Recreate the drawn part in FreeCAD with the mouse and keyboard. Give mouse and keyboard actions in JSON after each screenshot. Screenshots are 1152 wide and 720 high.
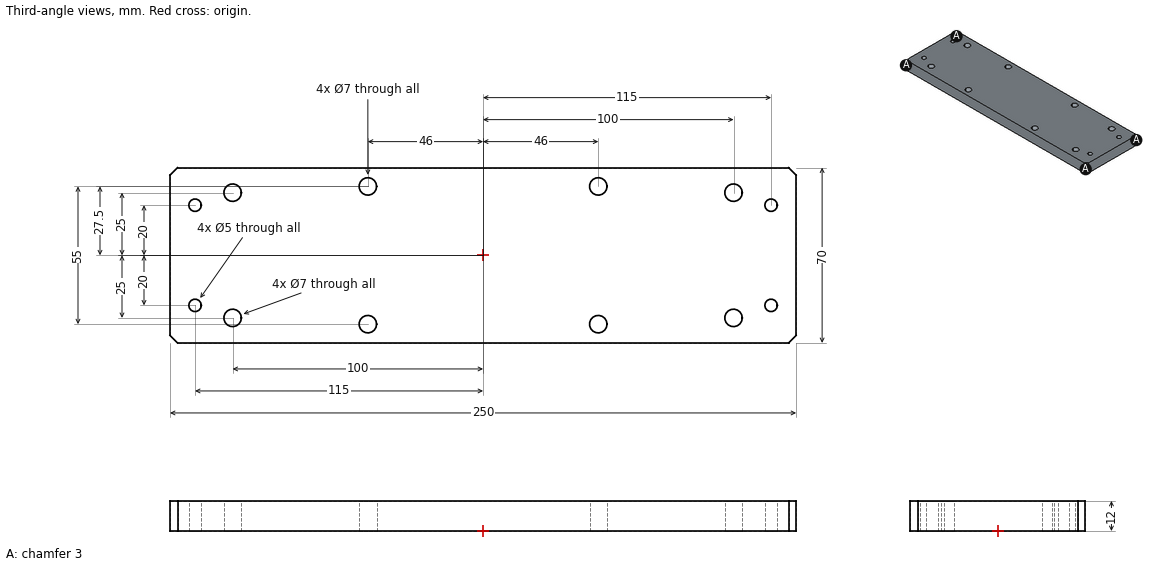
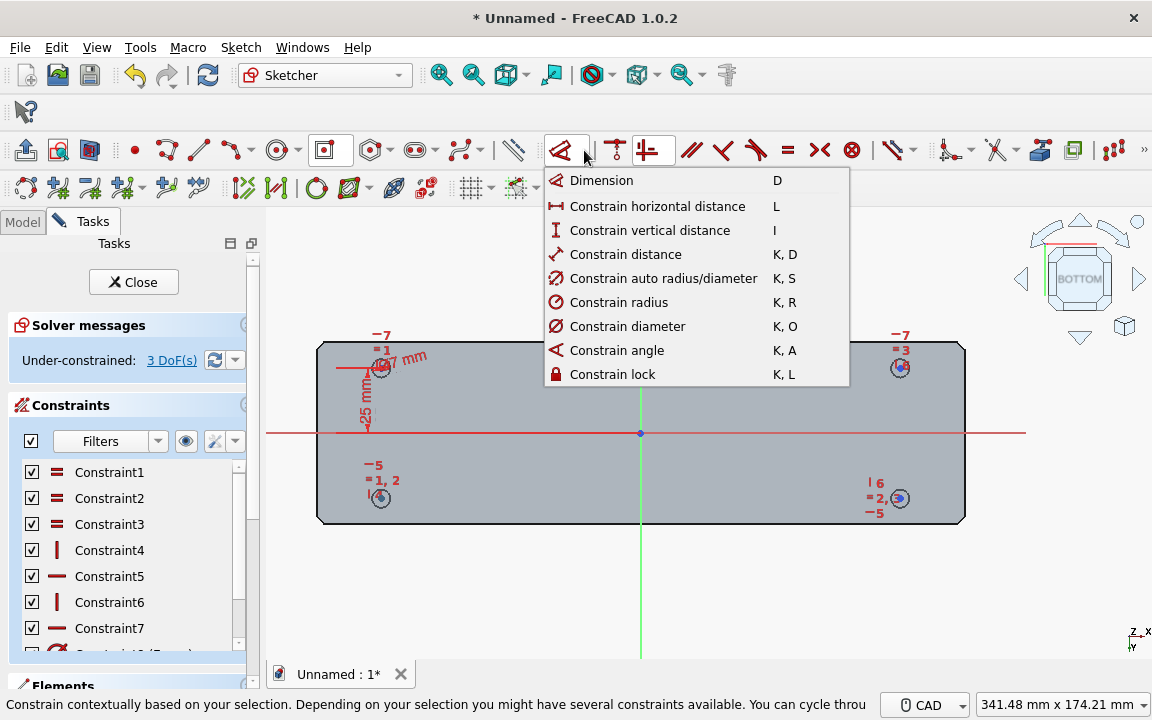
{"action": "left_click", "coordinate": [697, 230]}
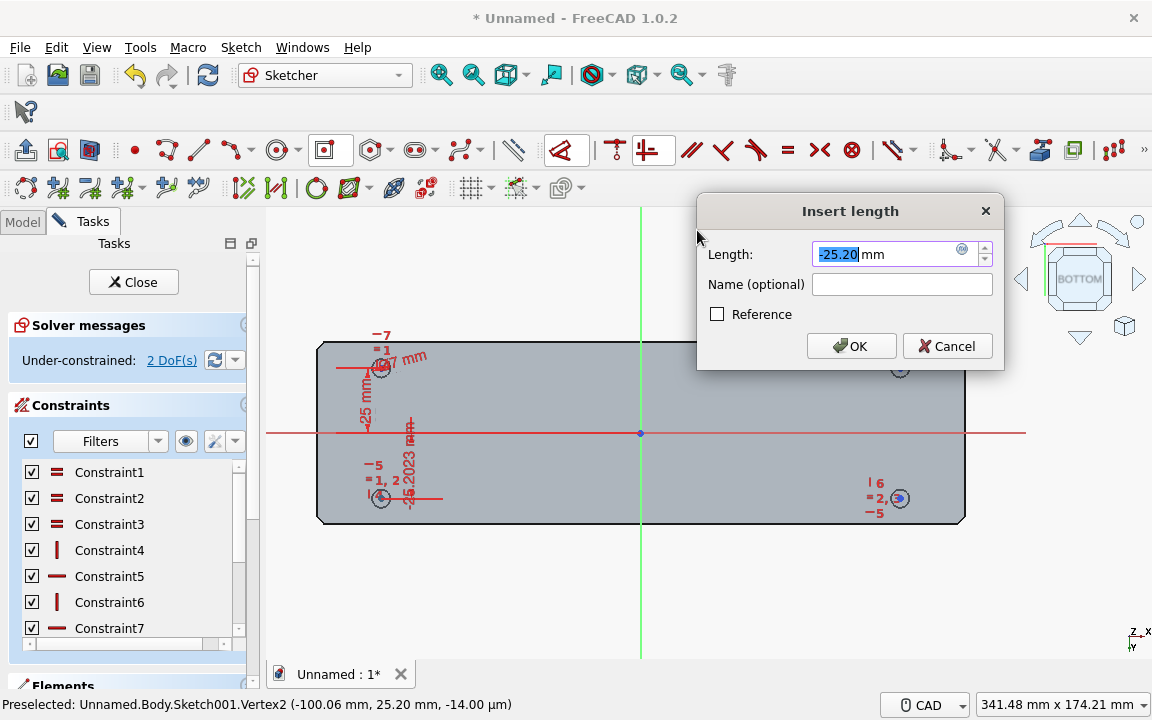
{"action": "type", "text": "-25"}
{"action": "key", "text": "Return"}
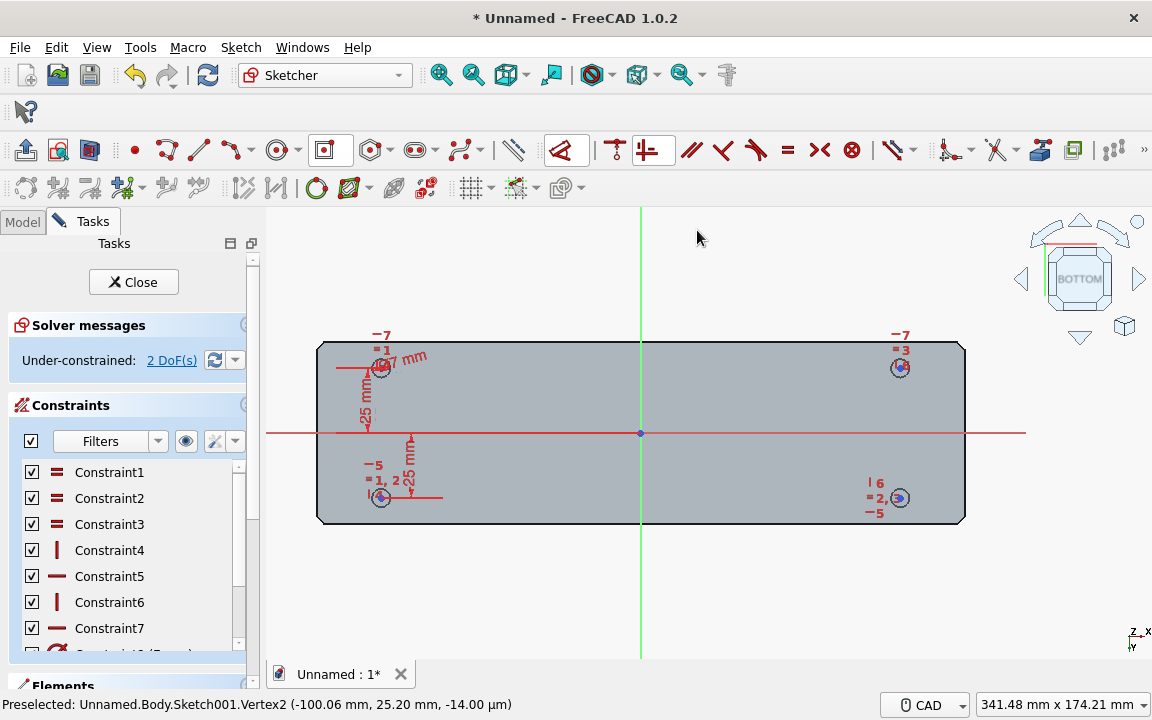
{"action": "left_click", "coordinate": [381, 368]}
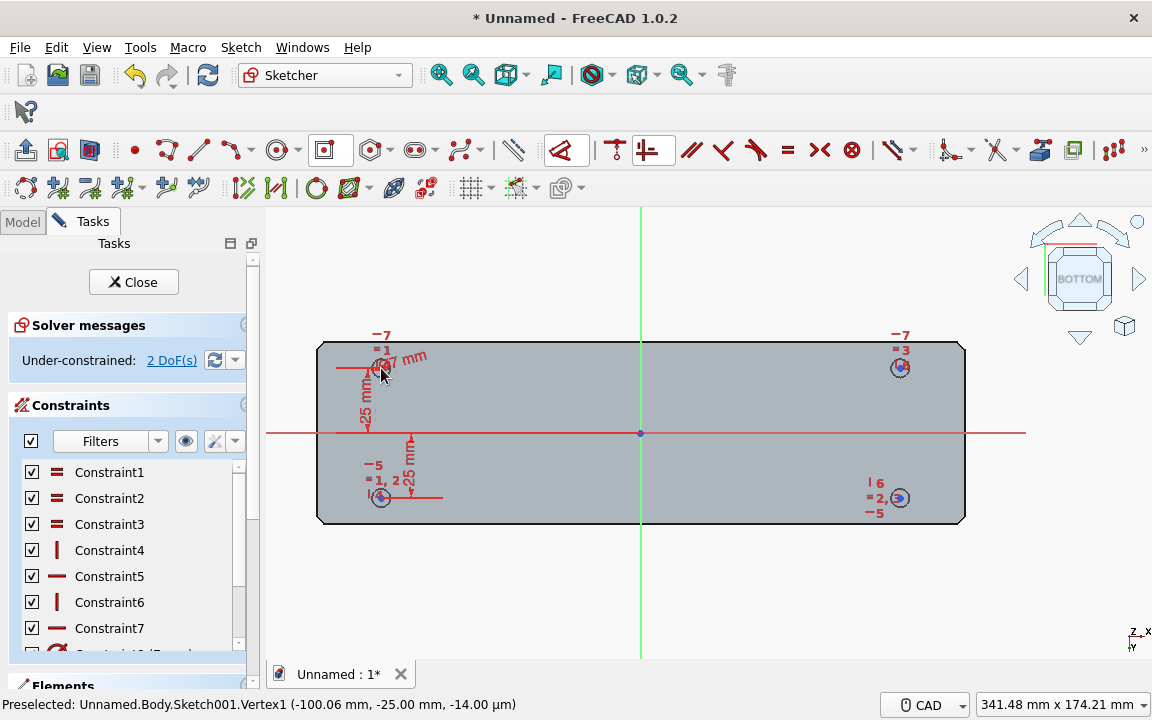
{"action": "left_click", "coordinate": [584, 150]}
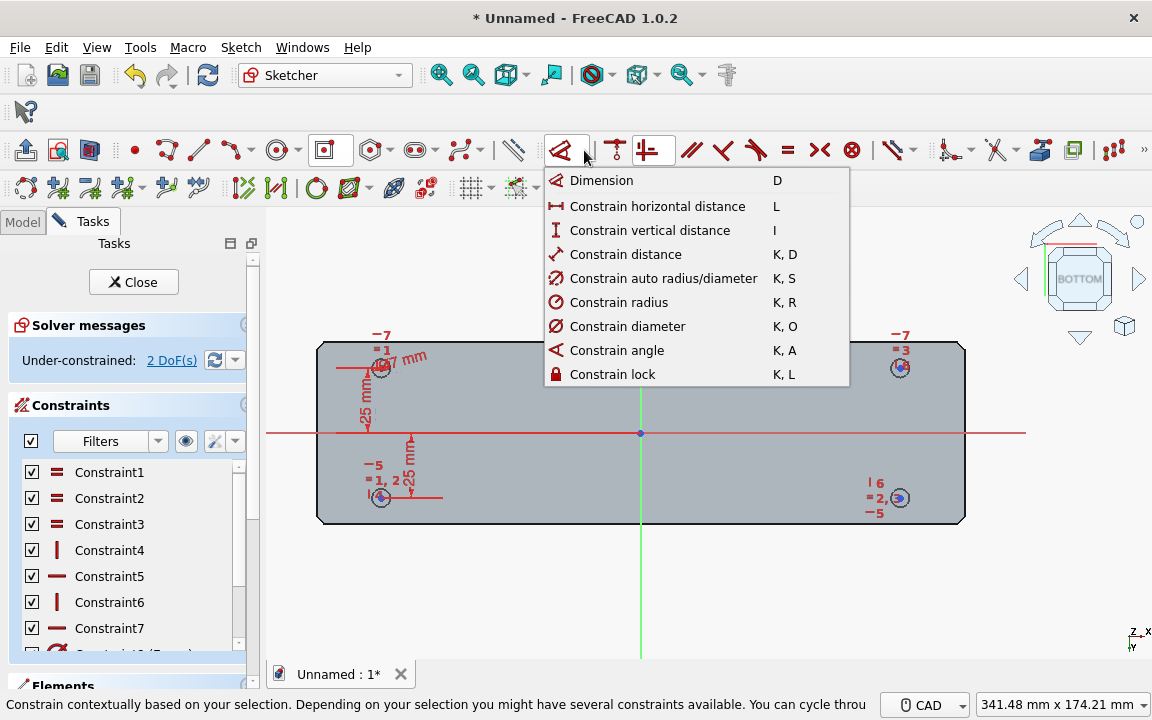
{"action": "left_click", "coordinate": [697, 206]}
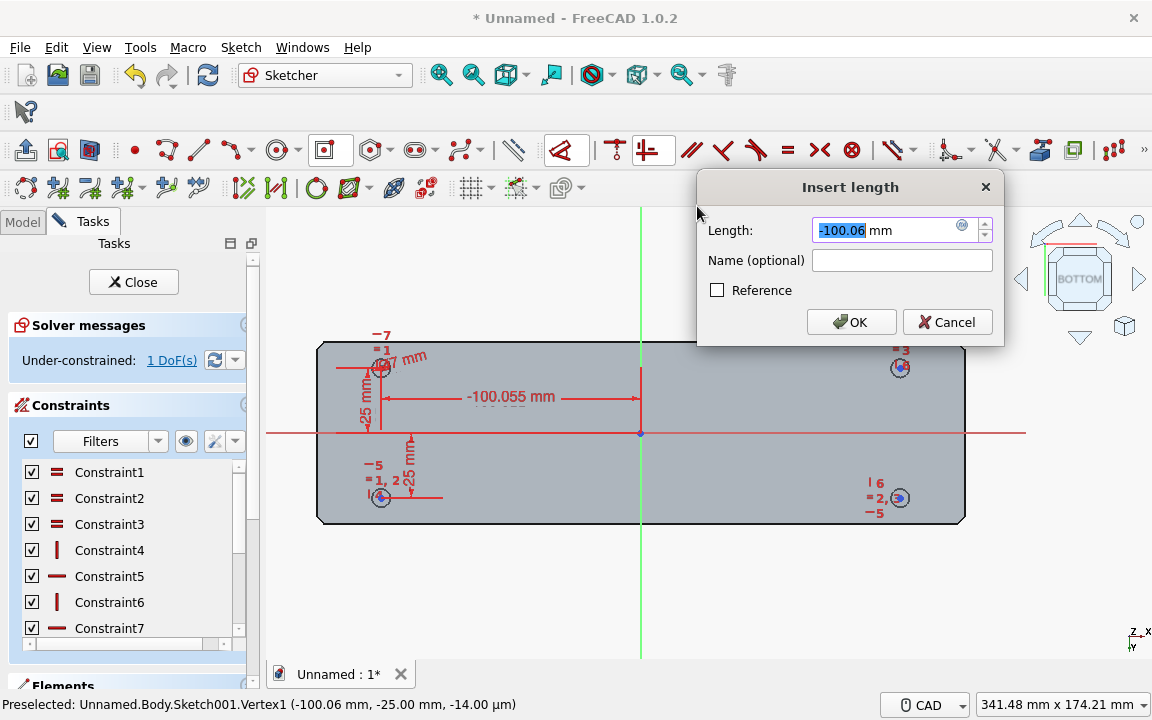
{"action": "type", "text": "-100"}
{"action": "key", "text": "Return"}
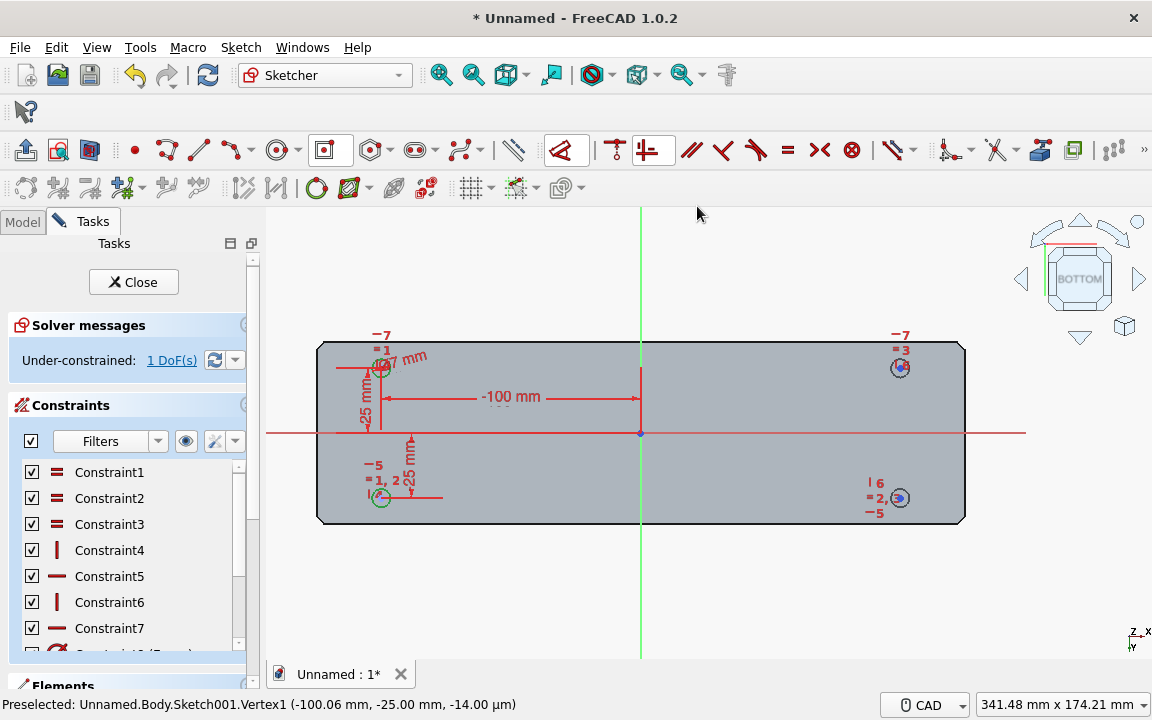
{"action": "left_click", "coordinate": [900, 498]}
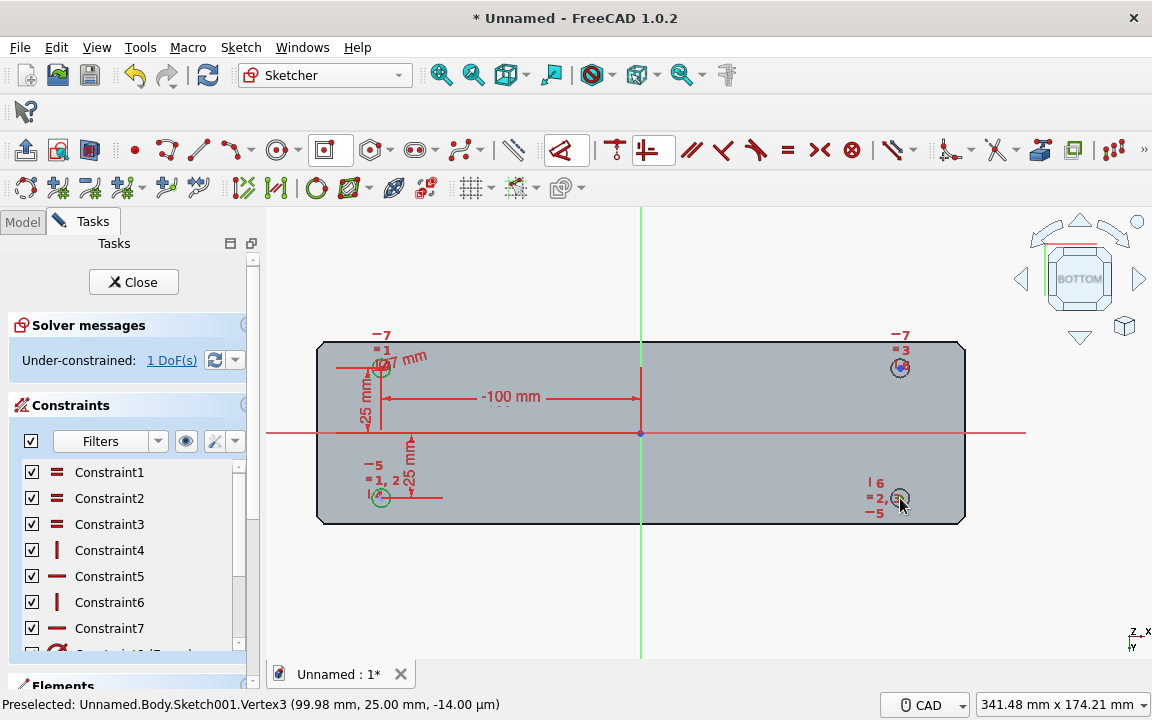
{"action": "key", "text": "l"}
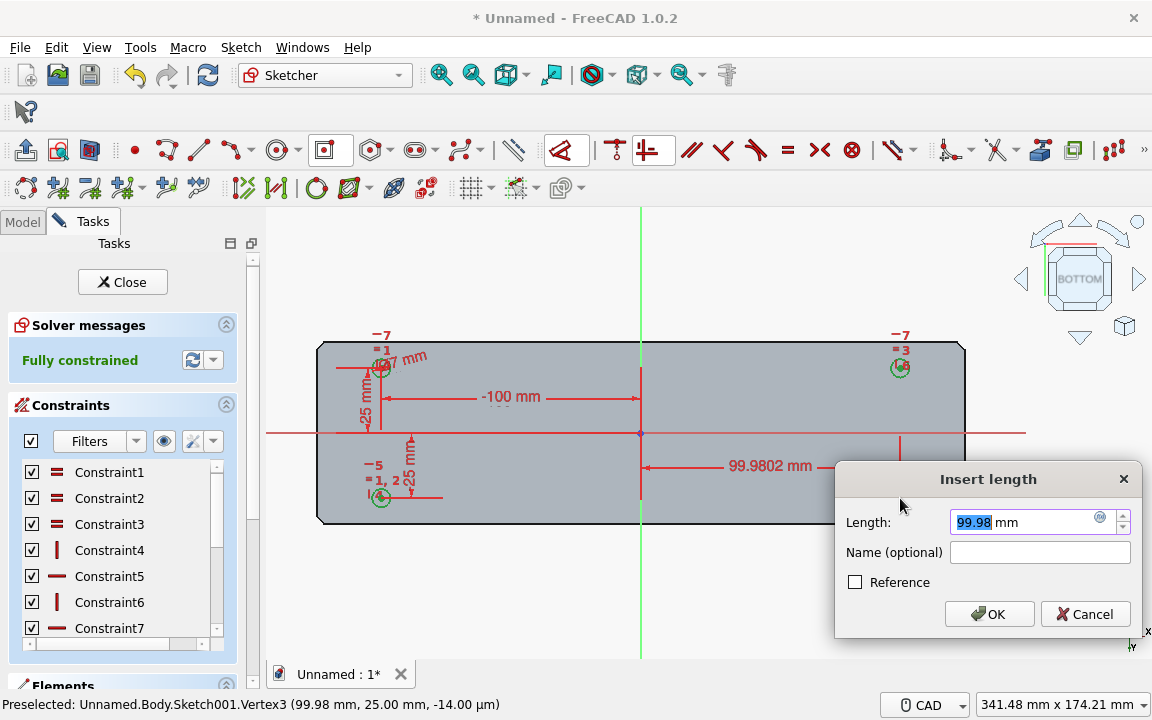
{"action": "type", "text": "100"}
{"action": "key", "text": "Return"}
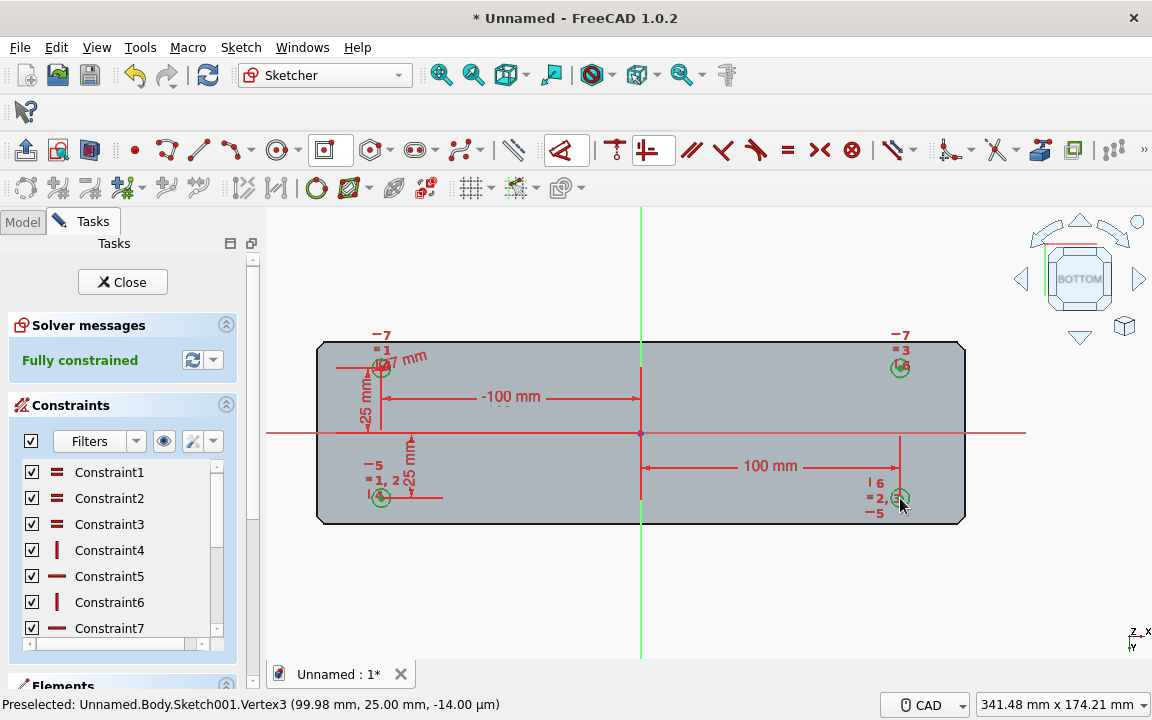
{"action": "left_click", "coordinate": [123, 282]}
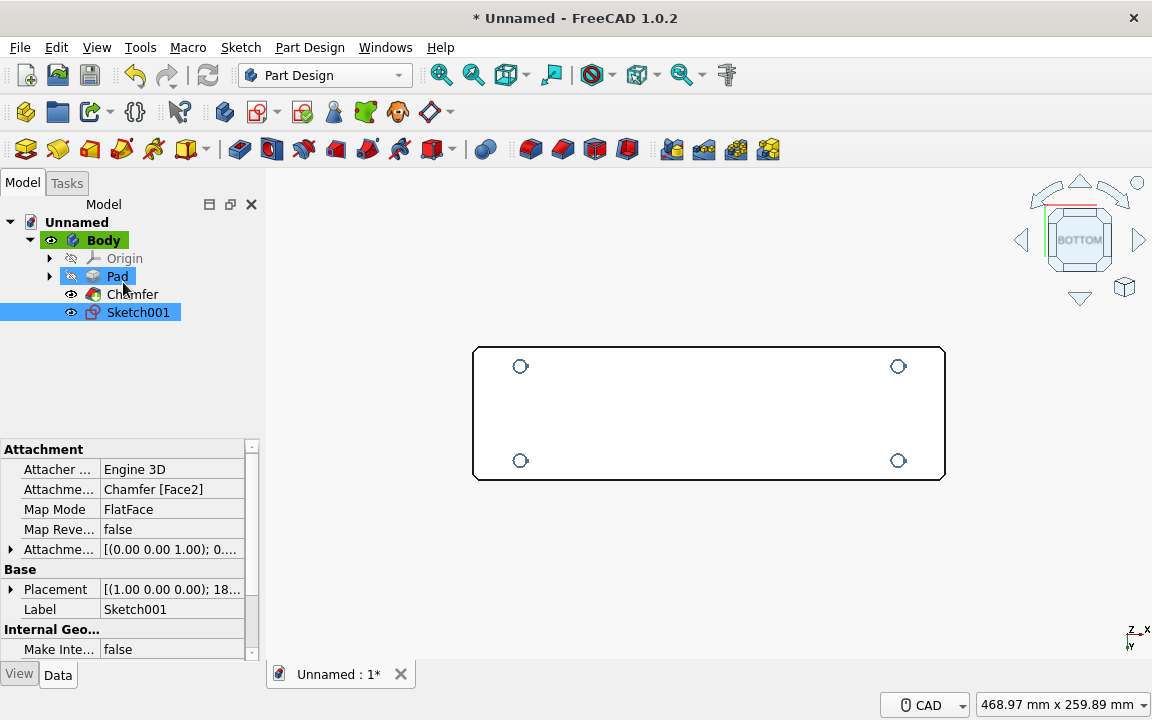
{"action": "left_click", "coordinate": [272, 150]}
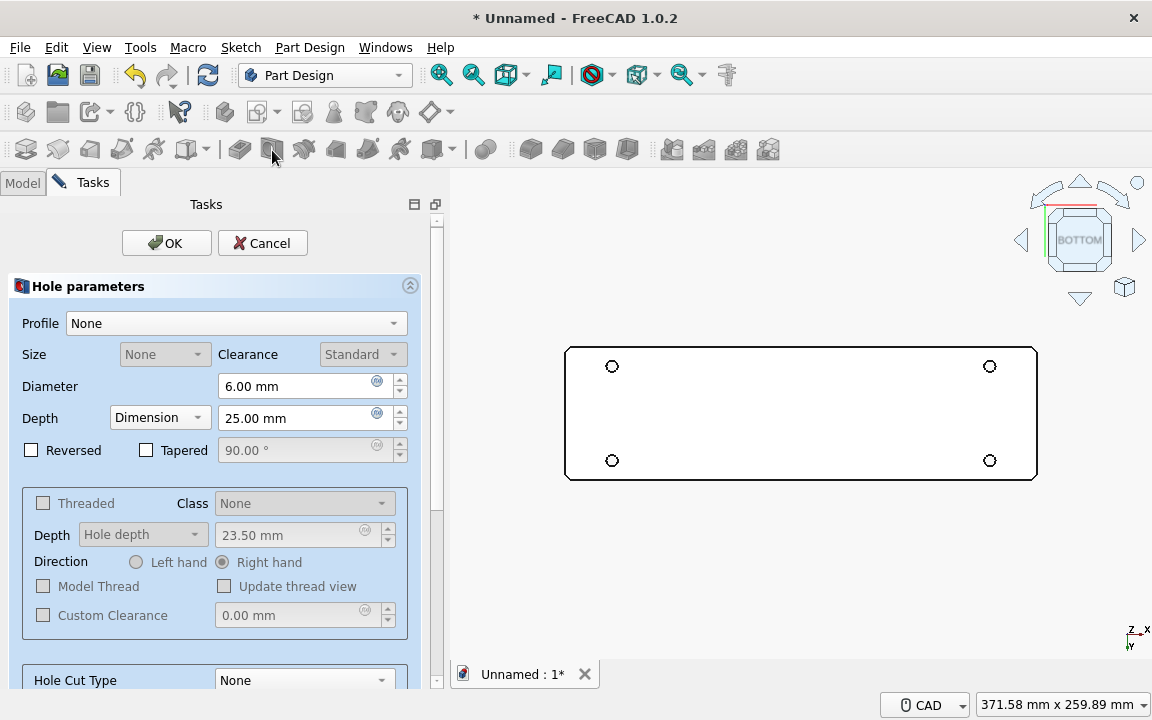
{"action": "triple_click", "coordinate": [305, 386]}